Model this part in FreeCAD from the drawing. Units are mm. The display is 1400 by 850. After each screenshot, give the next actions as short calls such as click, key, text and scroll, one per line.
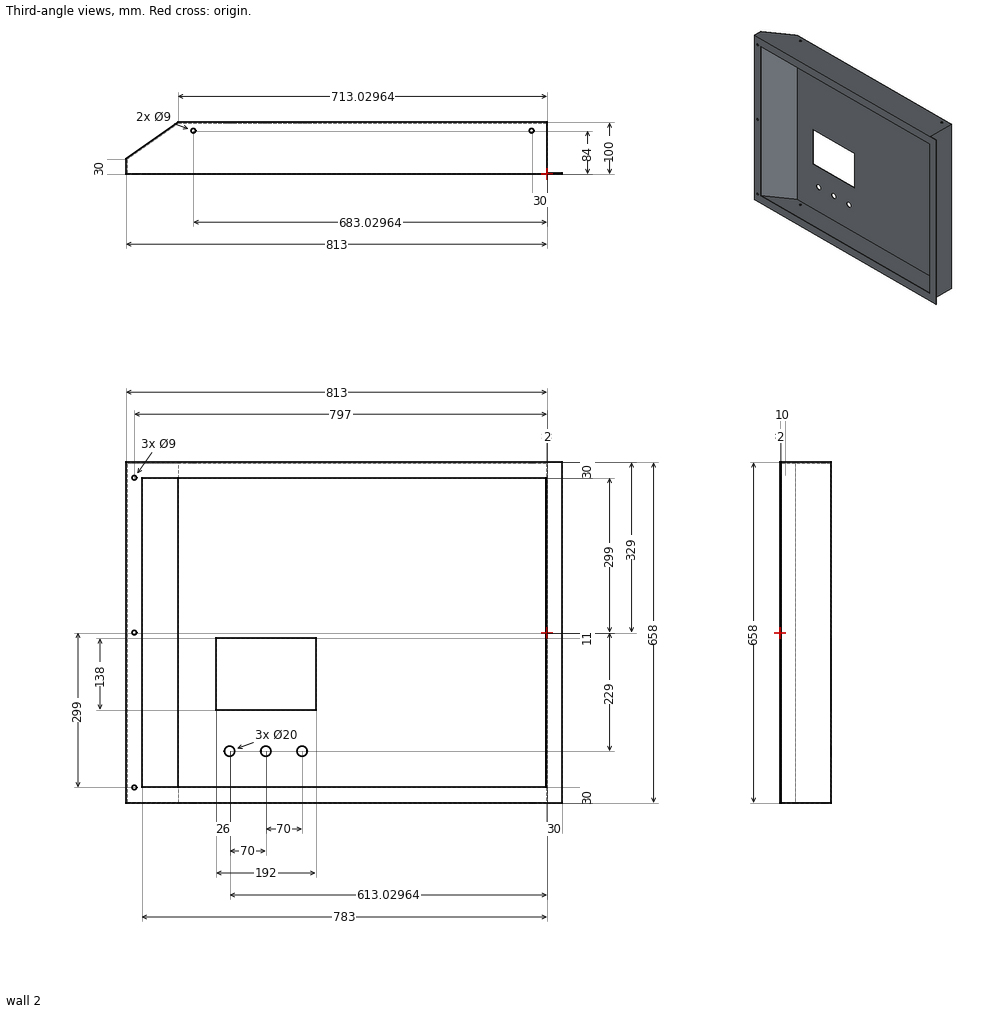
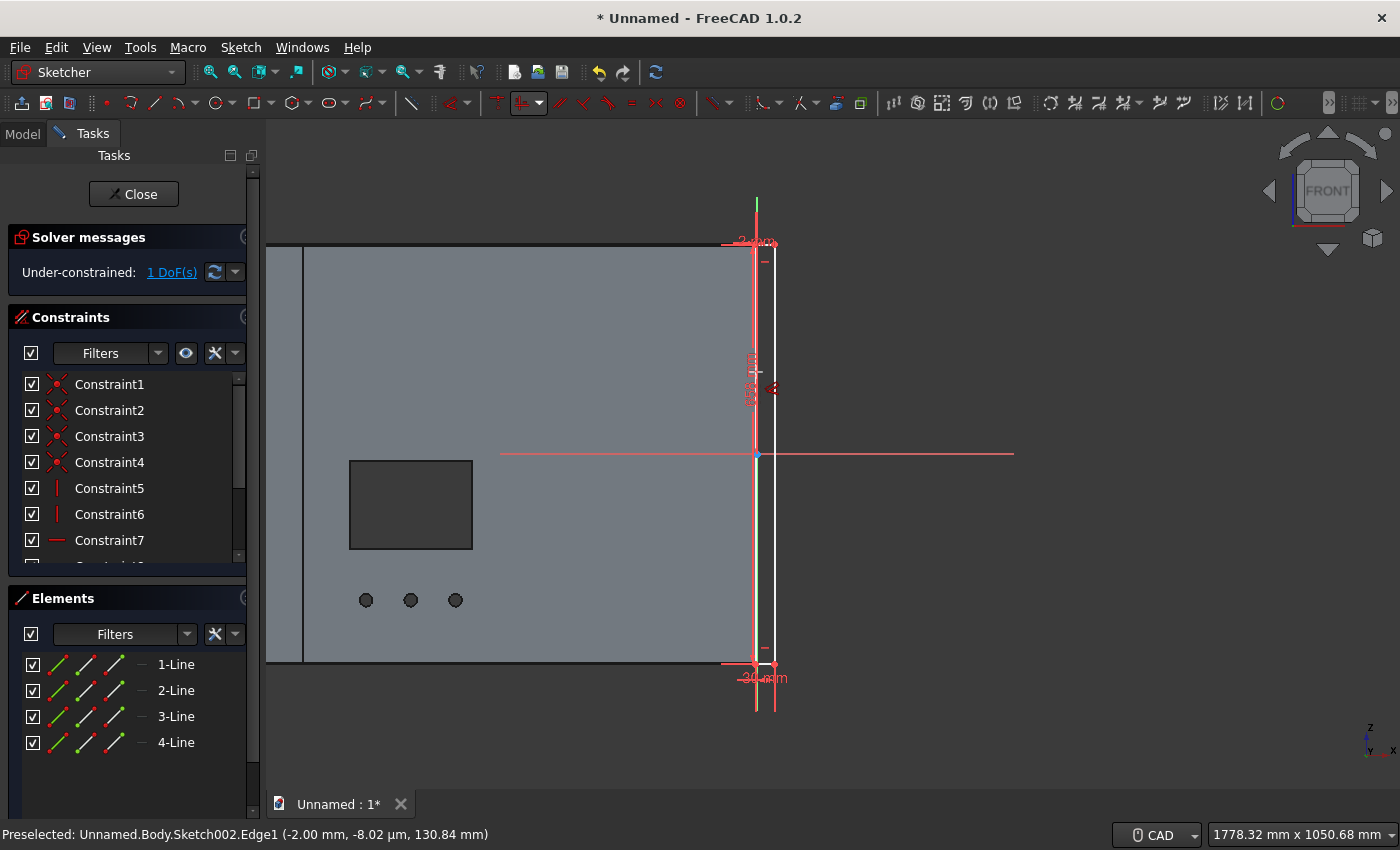
click(756, 245)
click(722, 350)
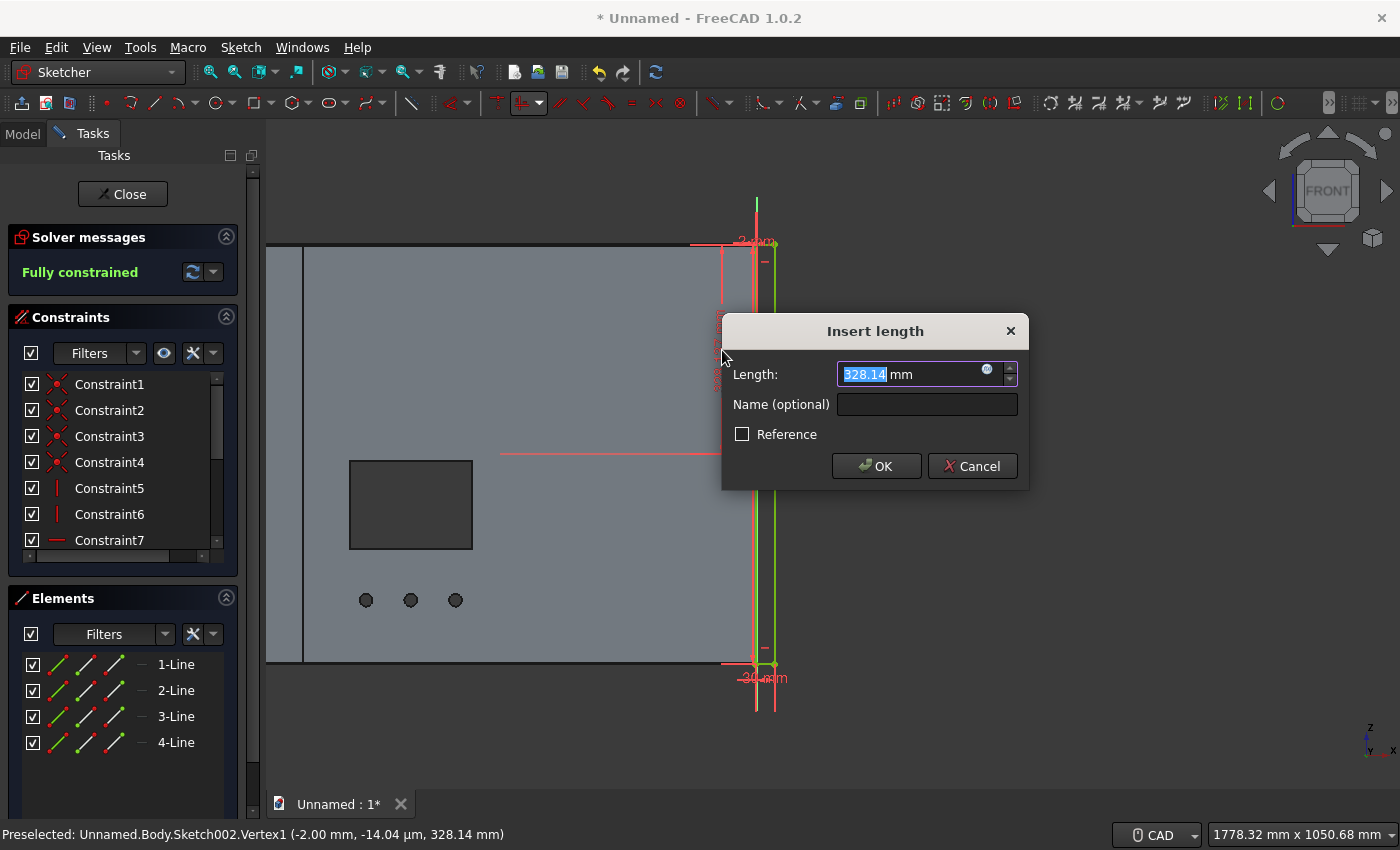
text(329)
key(Return)
key(Escape)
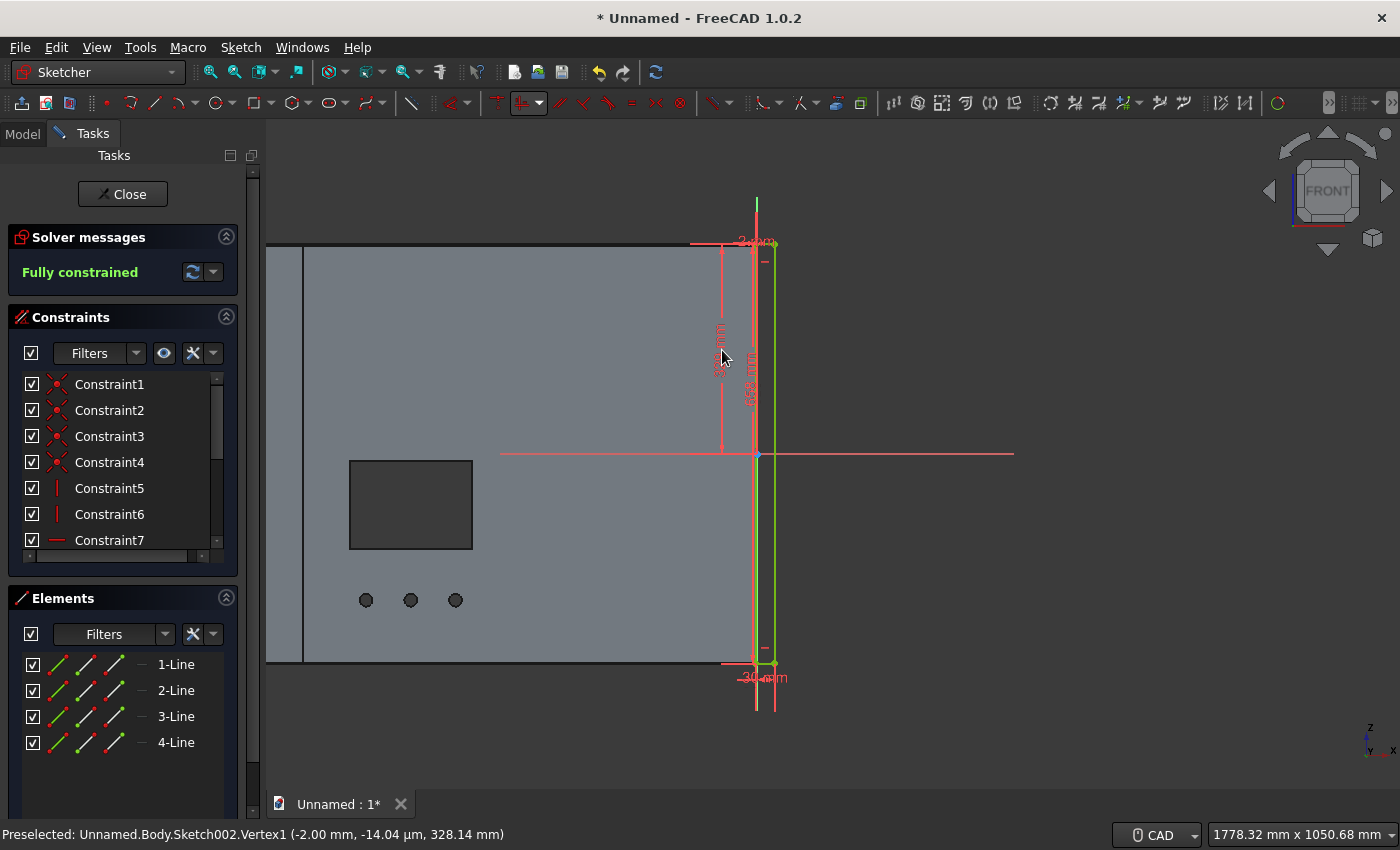
click(123, 194)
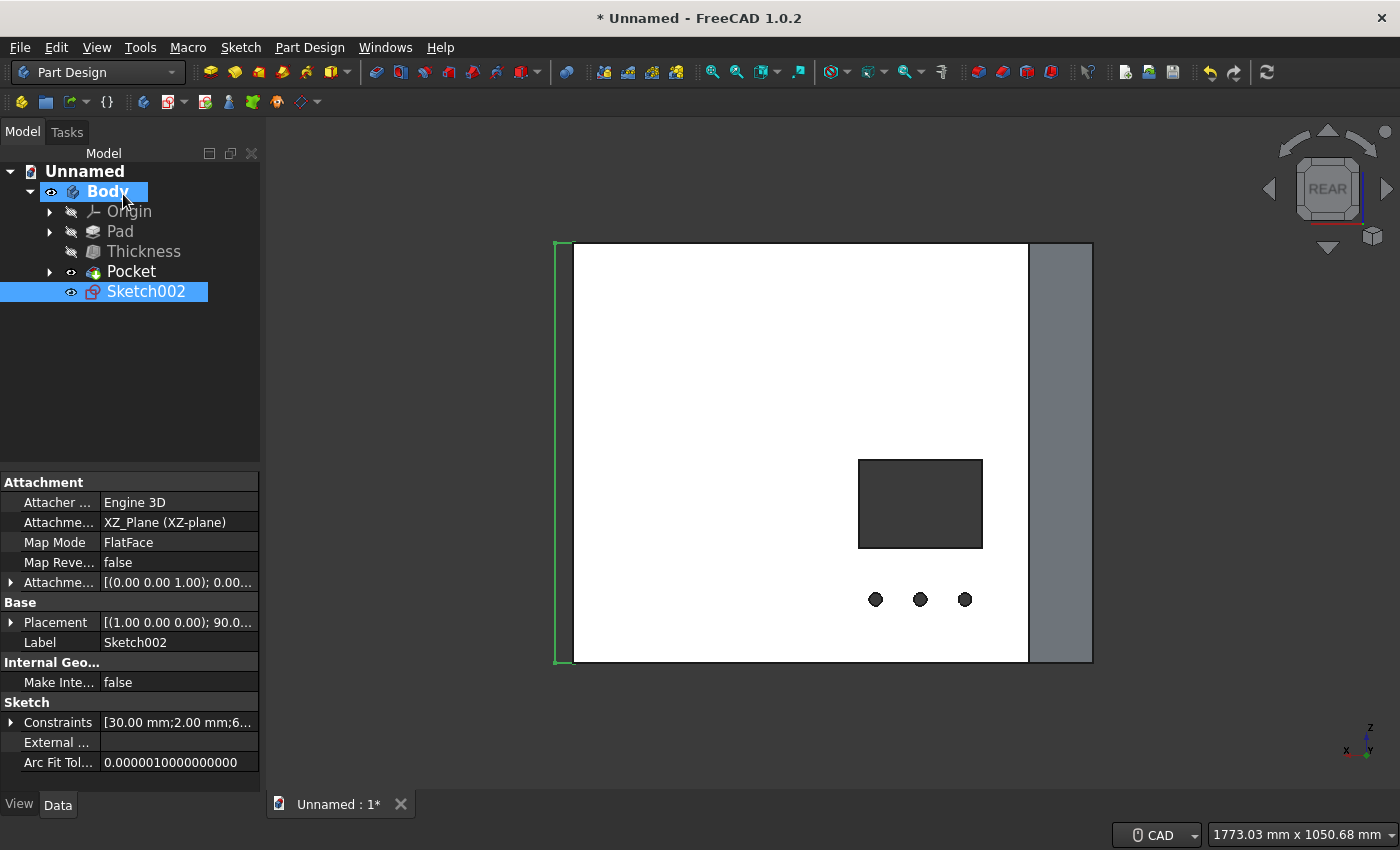
click(212, 72)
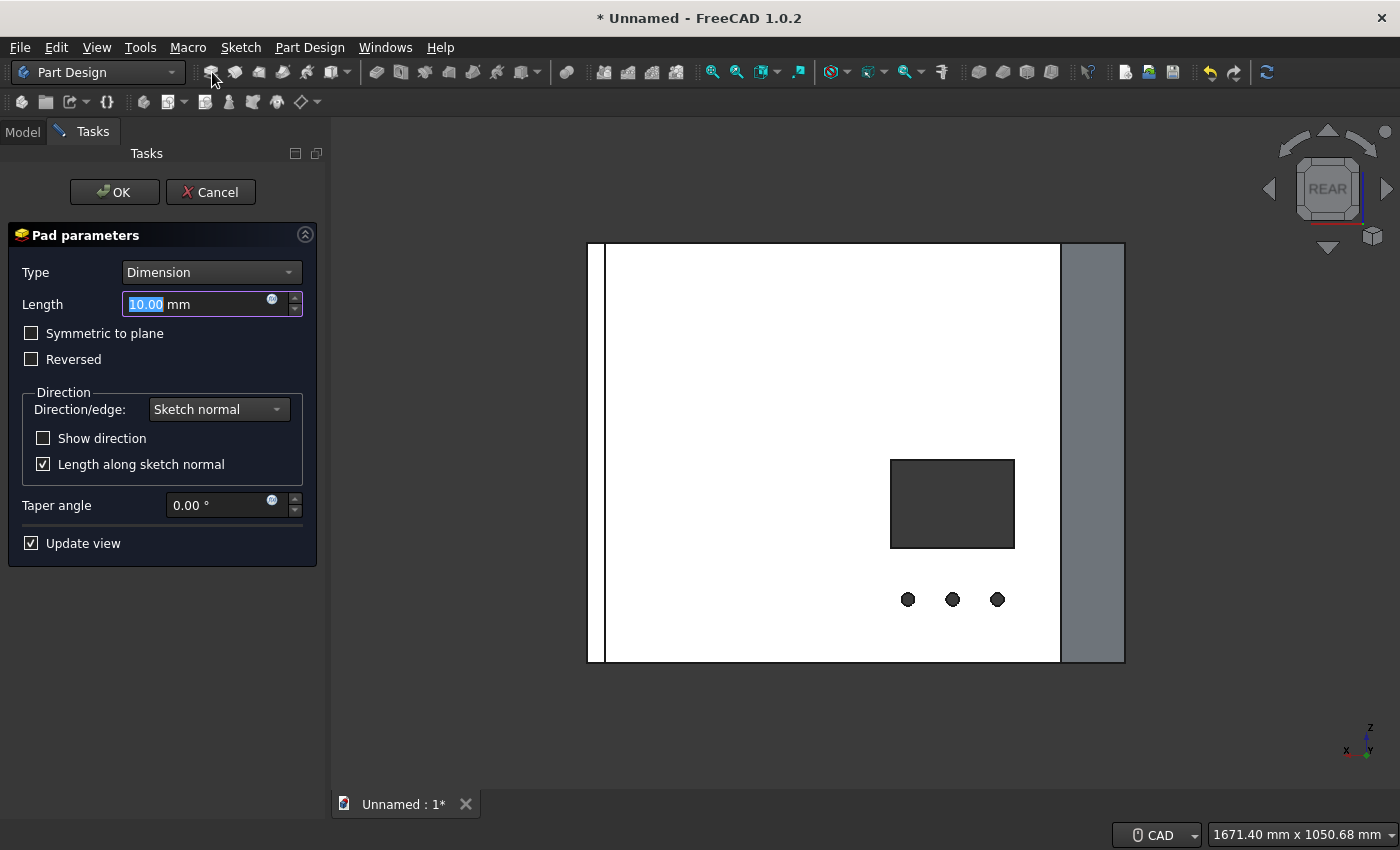
text(2)
key(Tab)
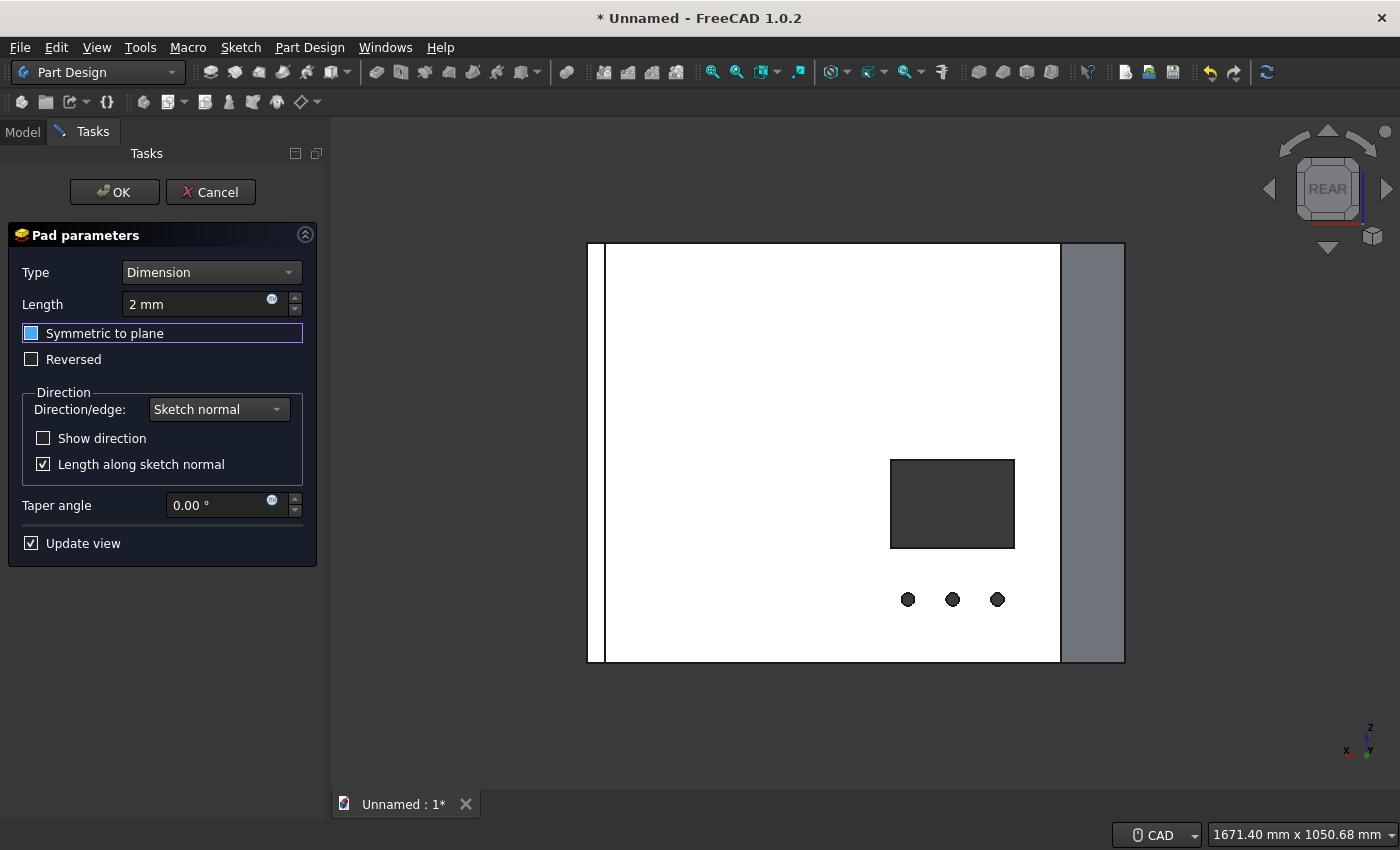
click(30, 359)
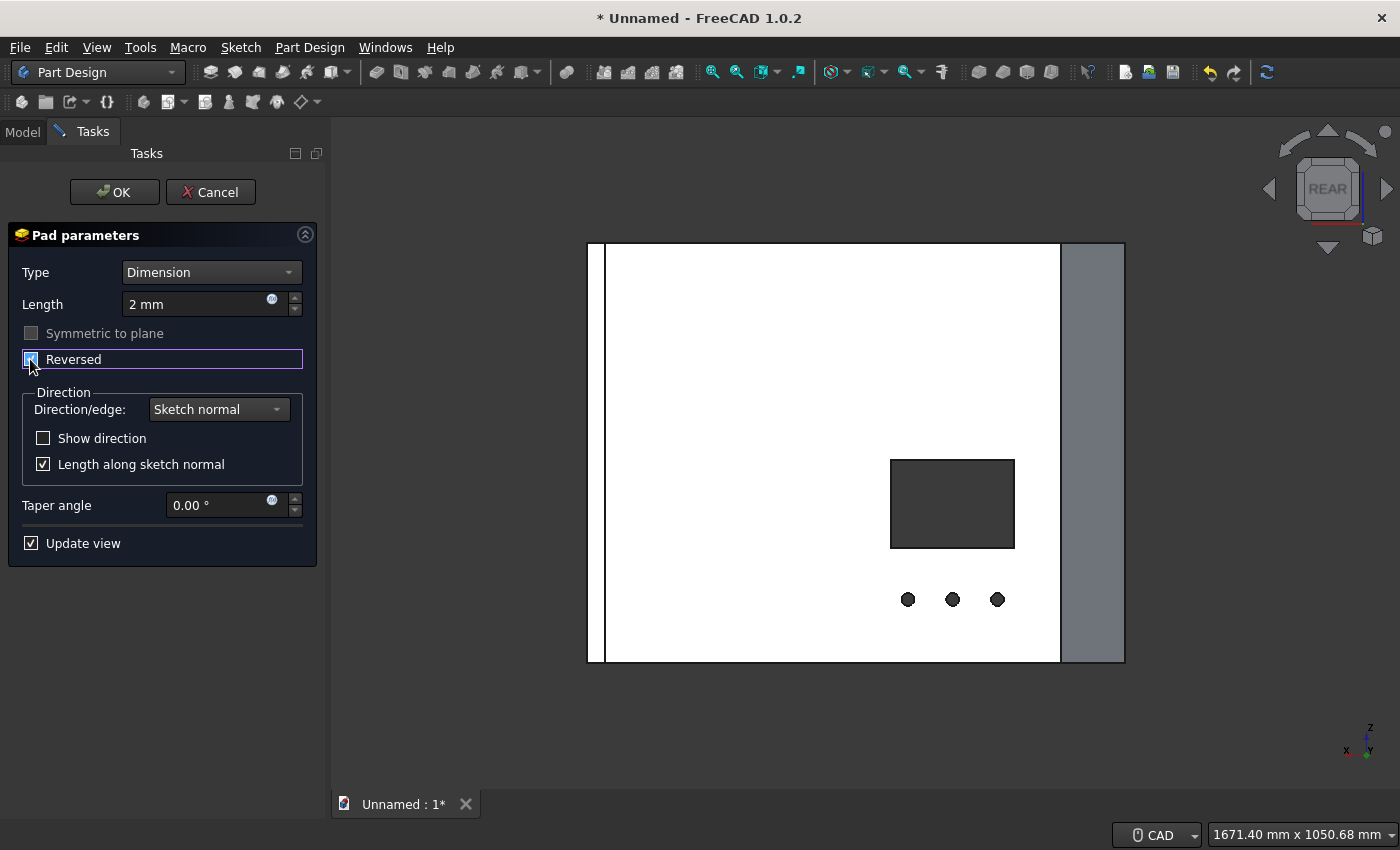
click(115, 192)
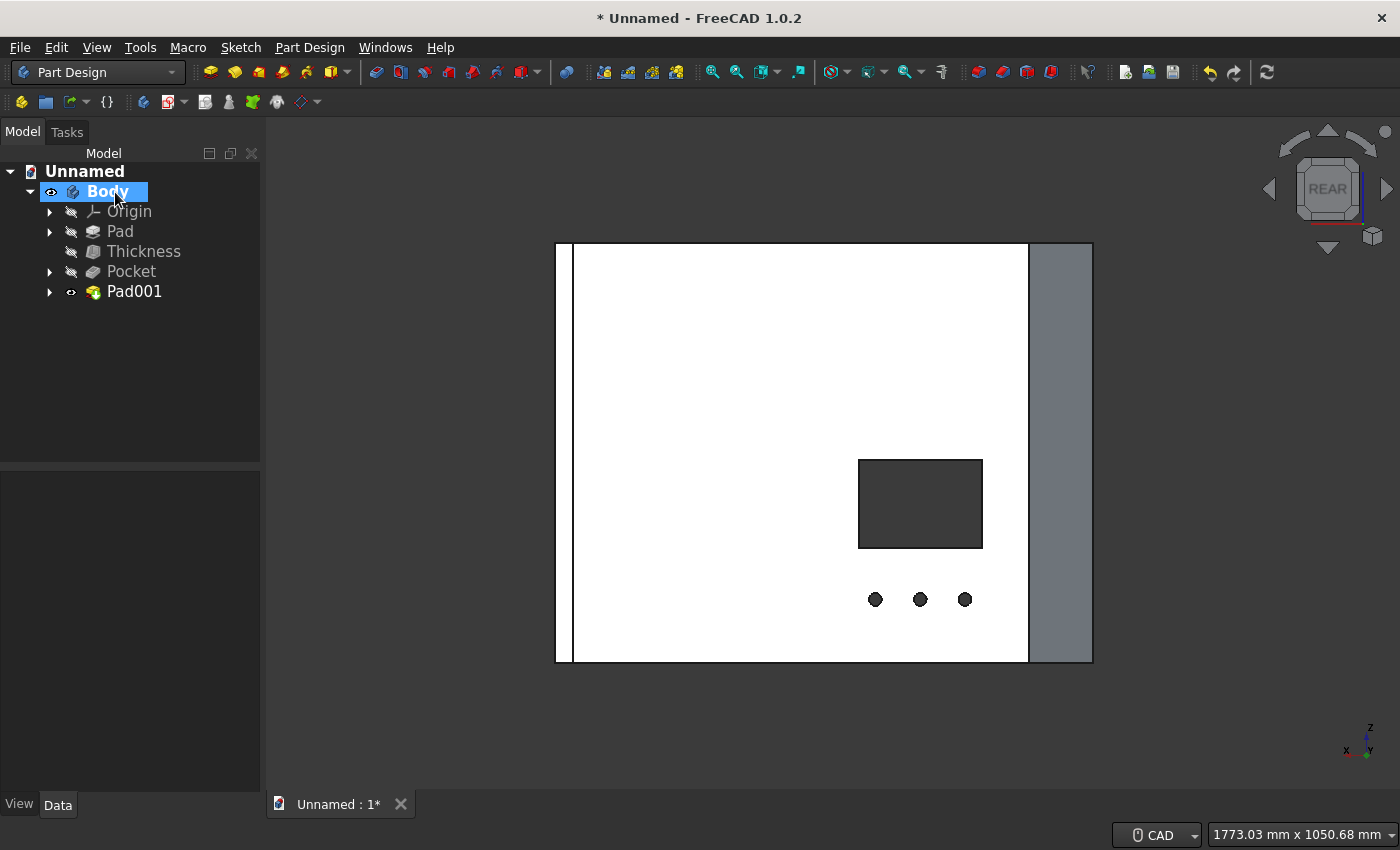
click(168, 102)